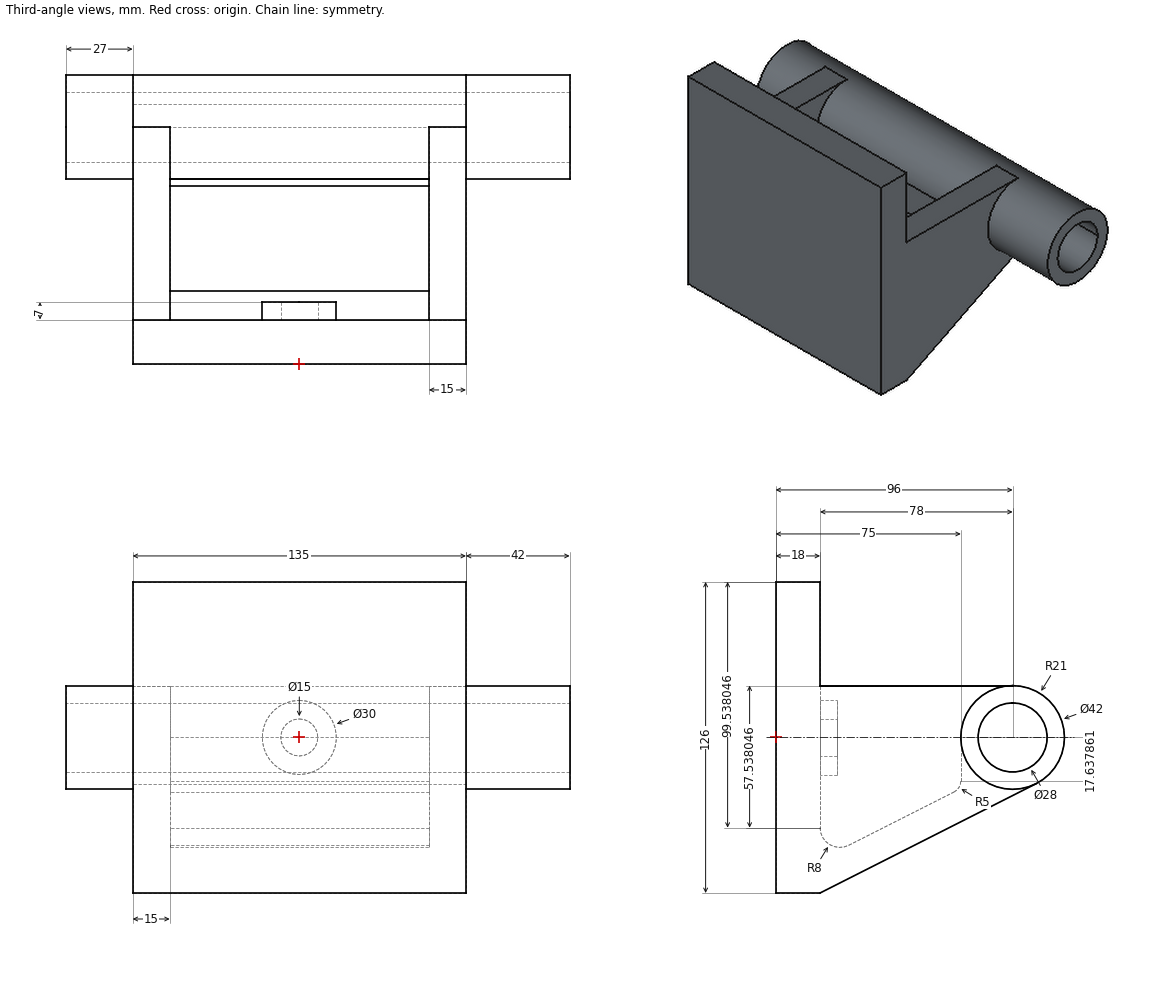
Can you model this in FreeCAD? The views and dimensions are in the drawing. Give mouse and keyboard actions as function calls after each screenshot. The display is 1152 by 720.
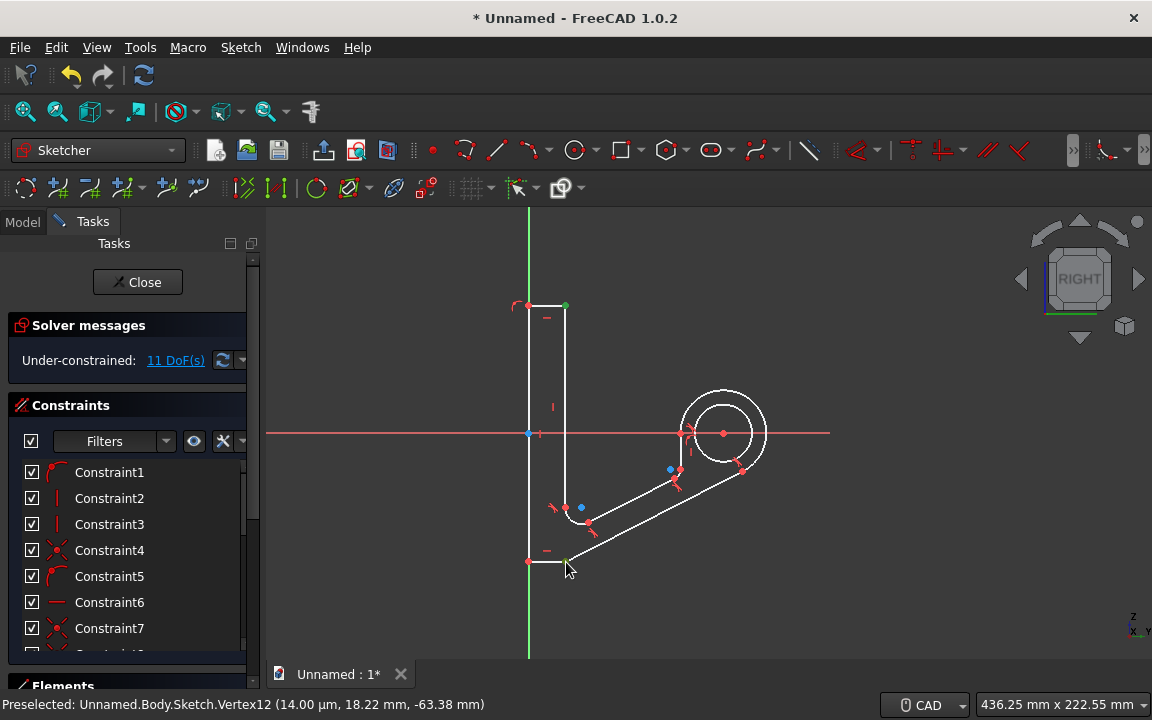
click(344, 433)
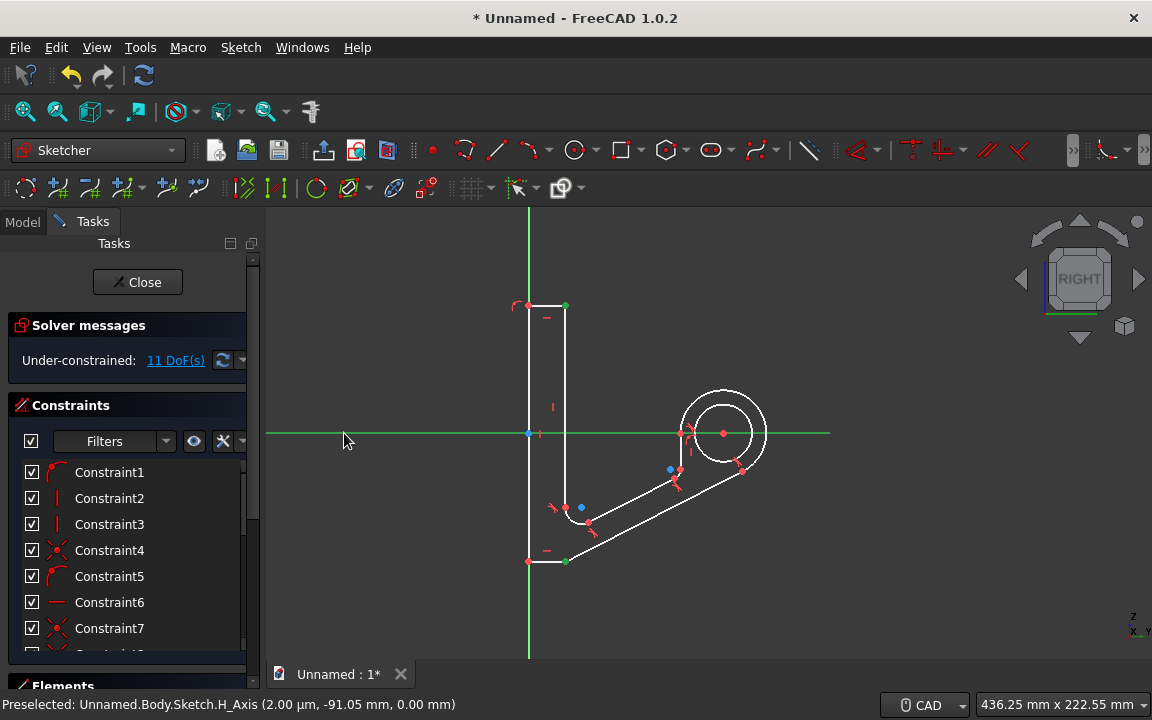
key(s)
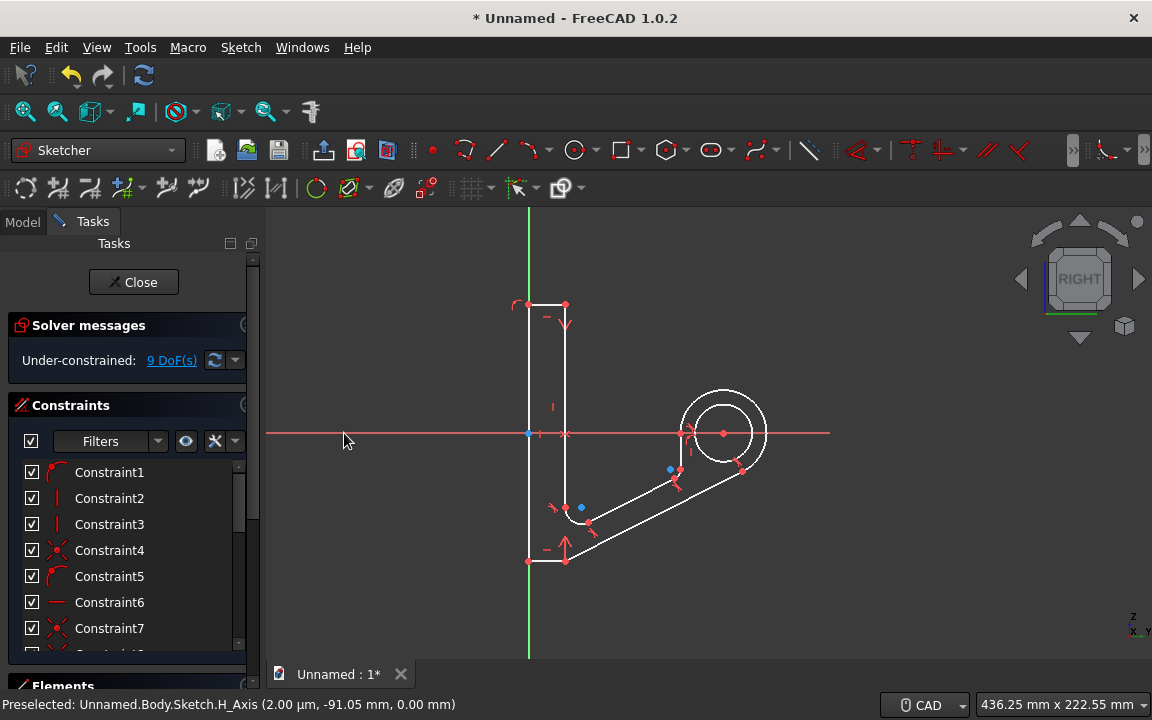
click(856, 150)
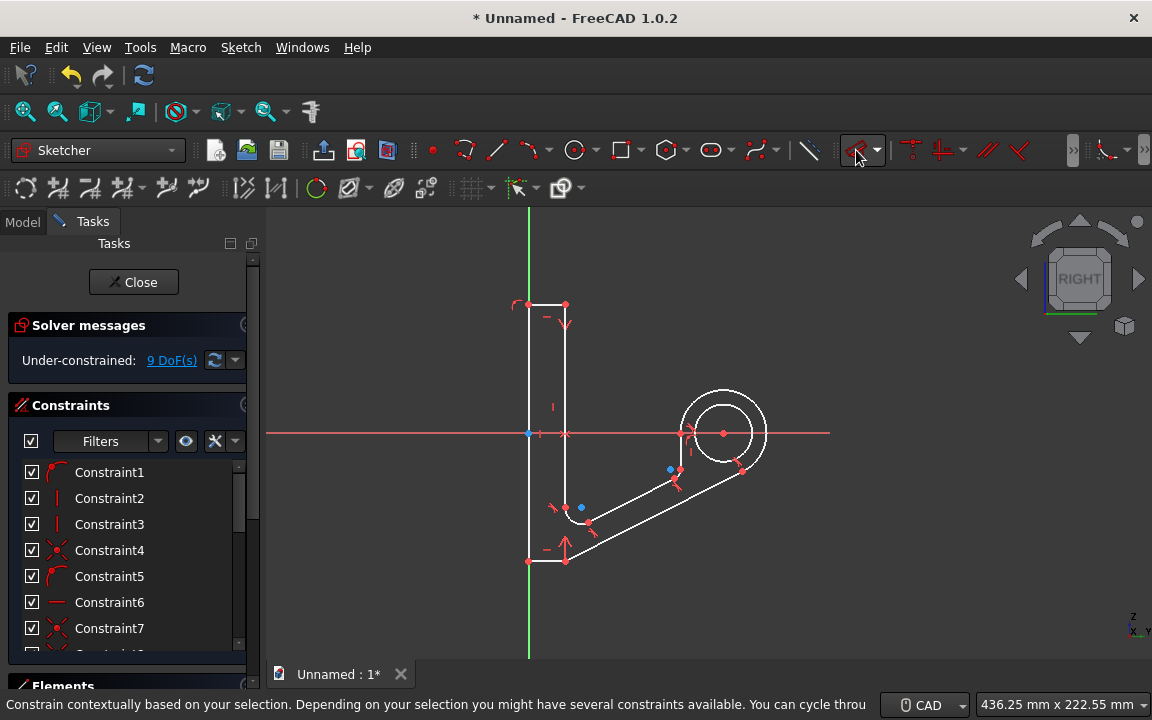
scroll(679, 475, up, 7)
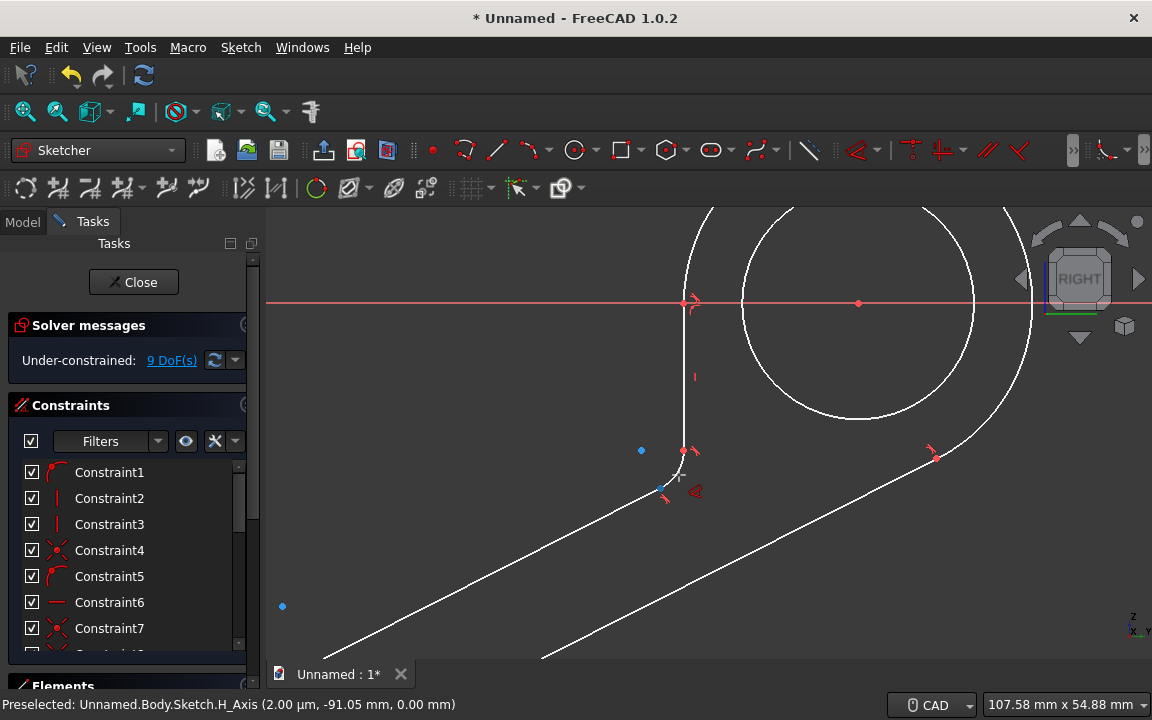
click(678, 472)
click(705, 488)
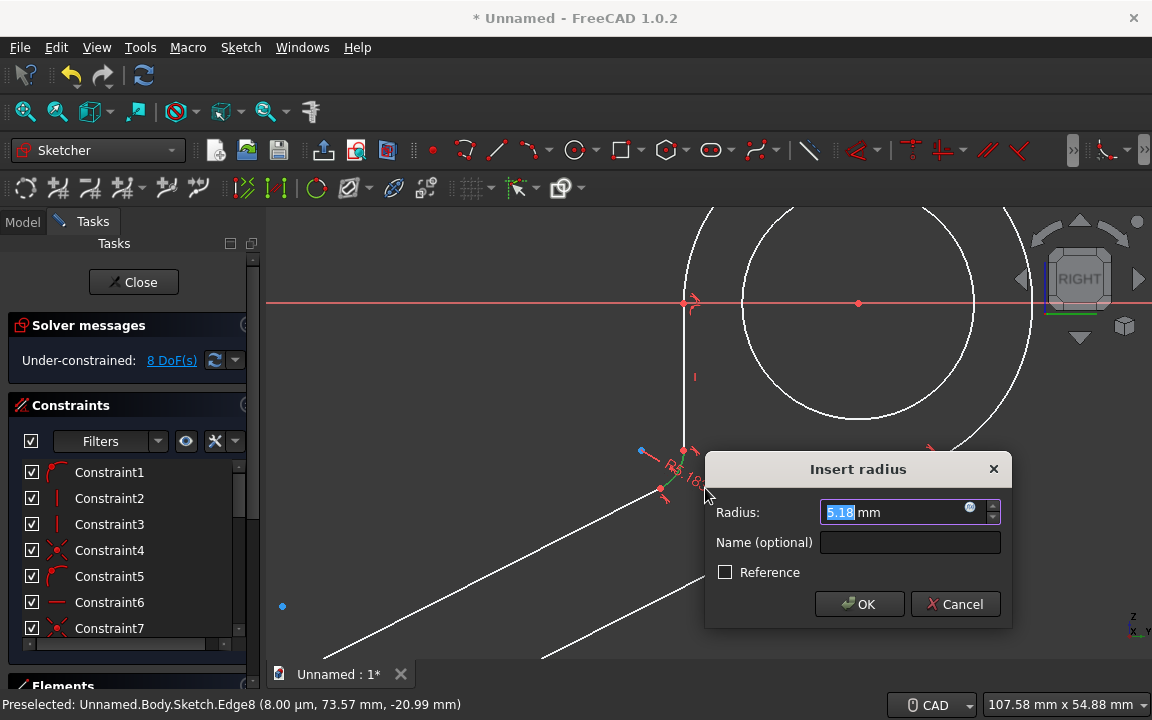
text(5)
key(Return)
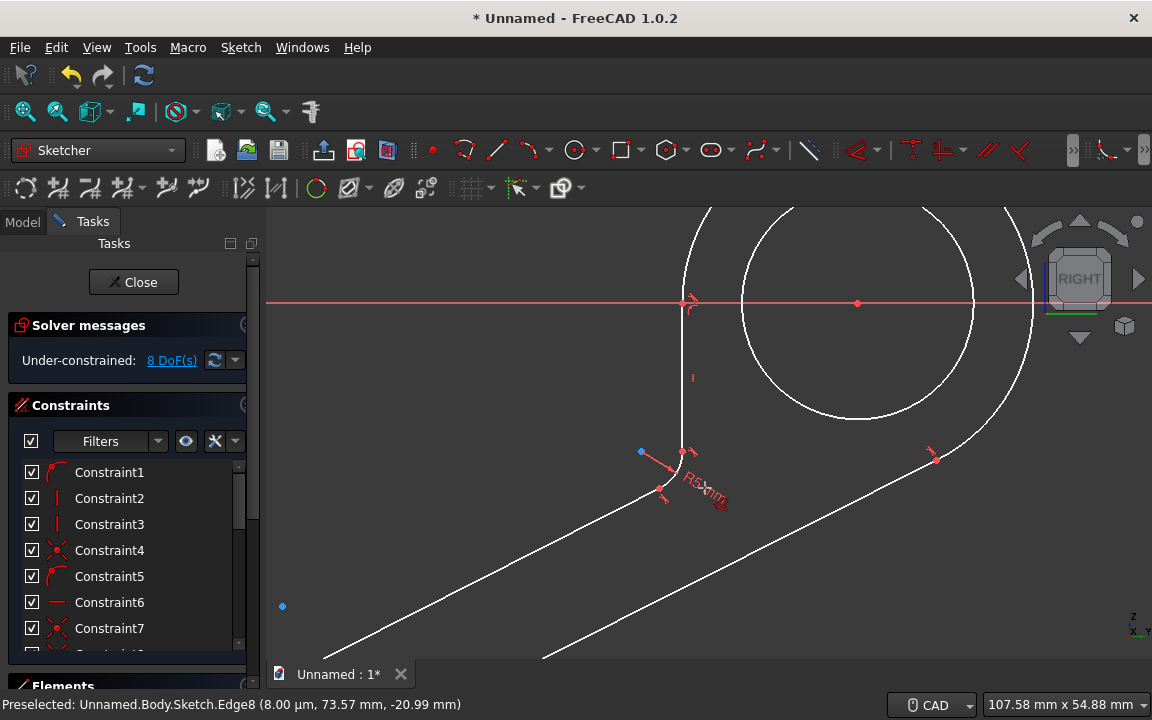
scroll(679, 475, down, 7)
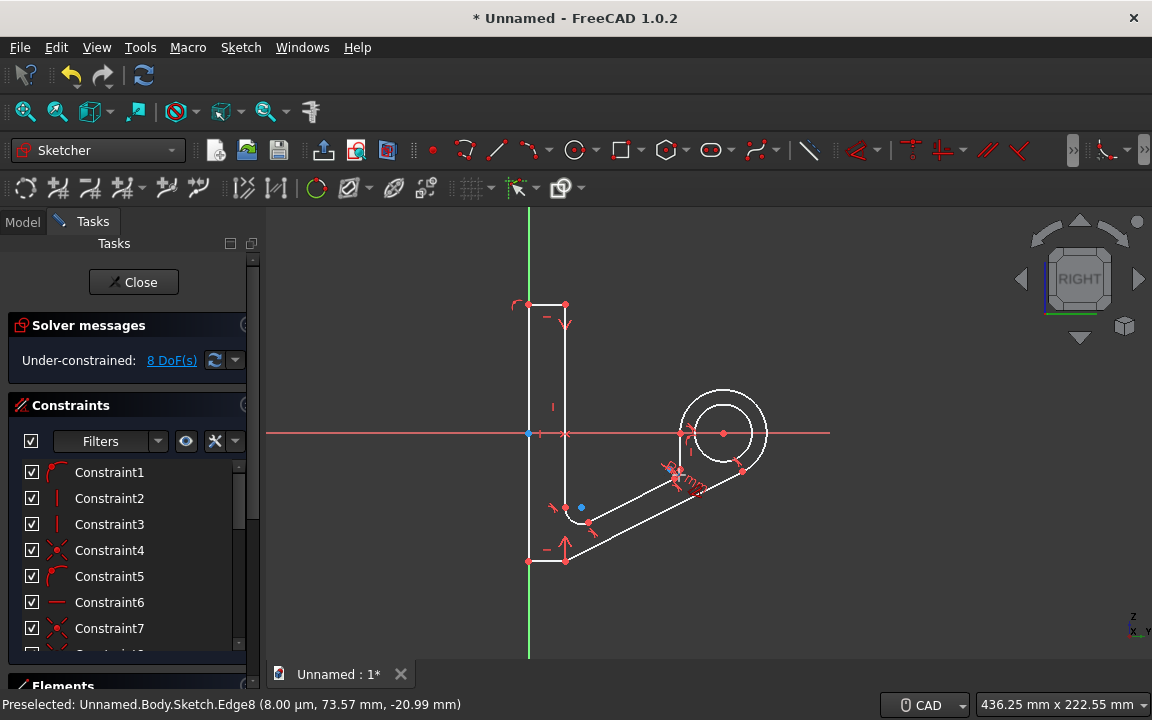
scroll(568, 517, up, 5)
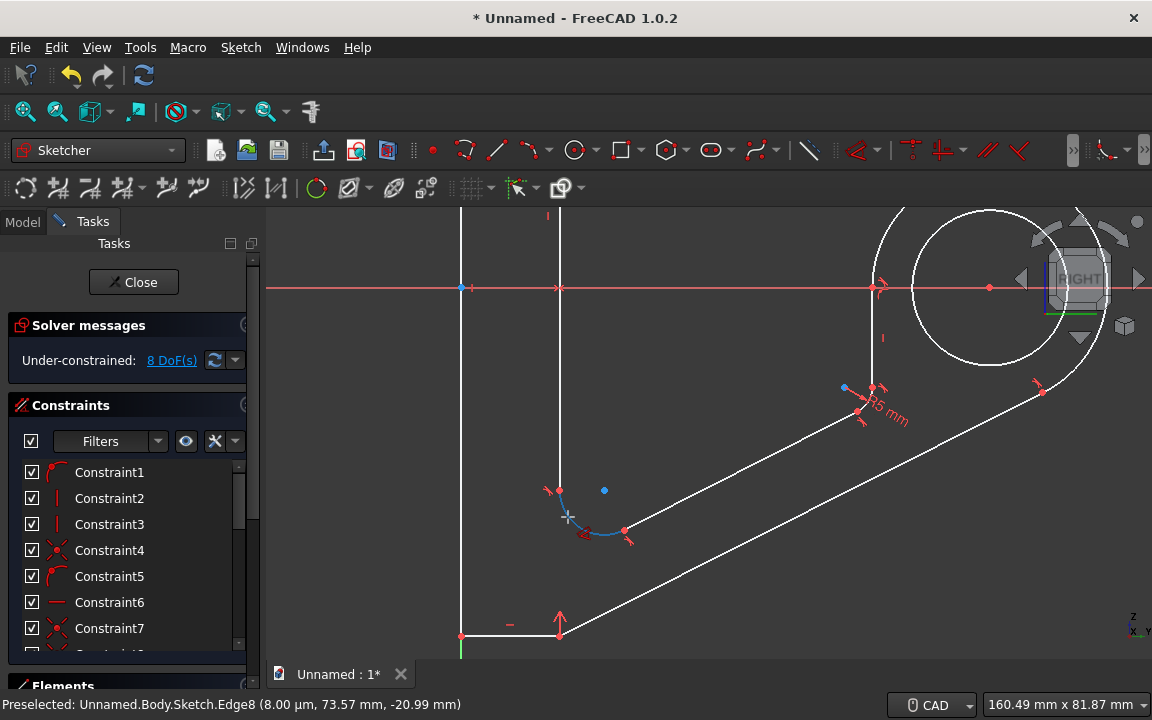
click(568, 516)
click(542, 534)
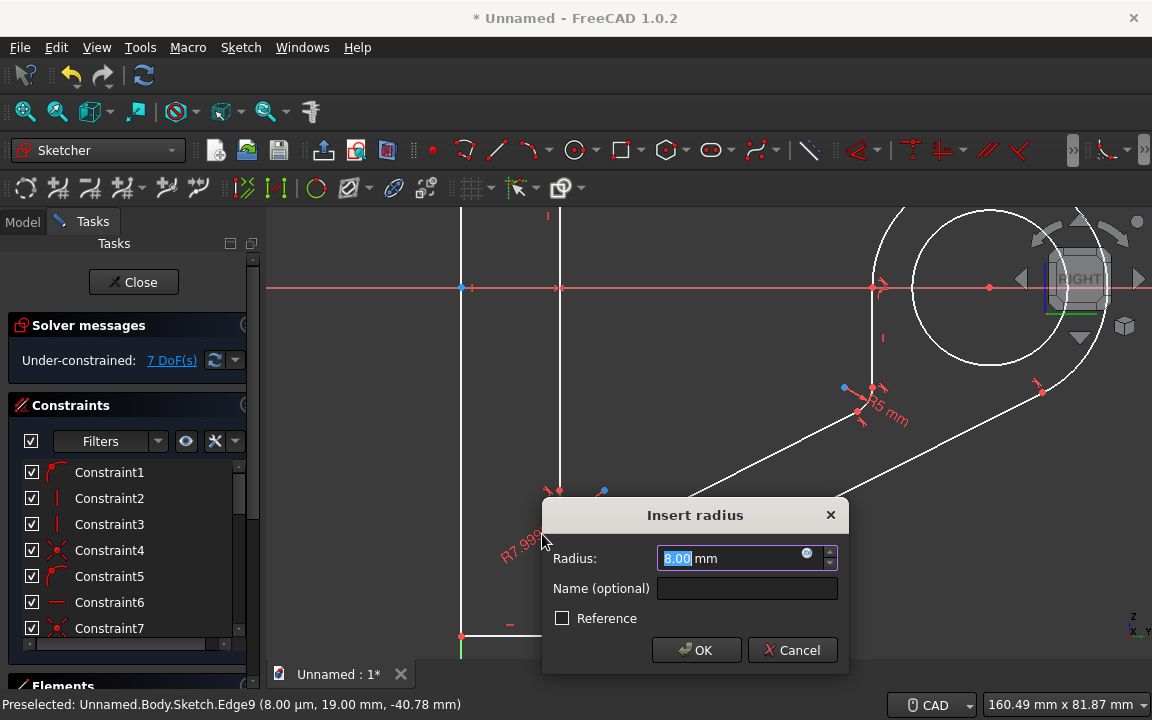
text(8)
key(Return)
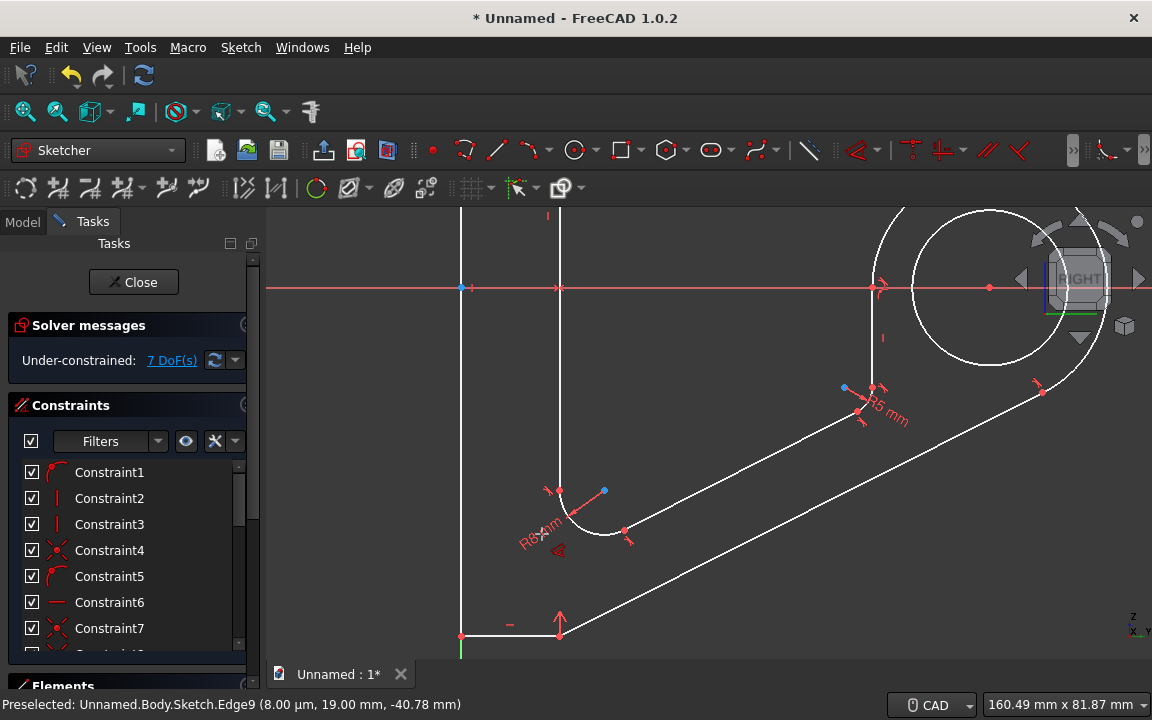
scroll(568, 517, down, 5)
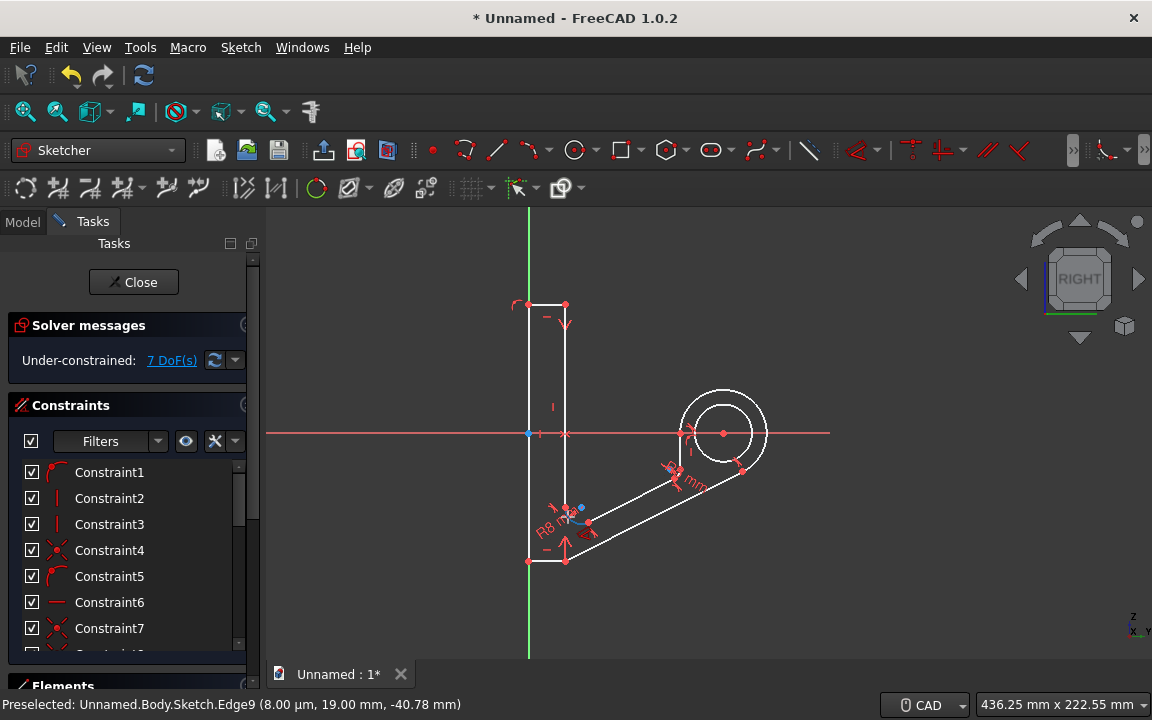
scroll(766, 426, up, 4)